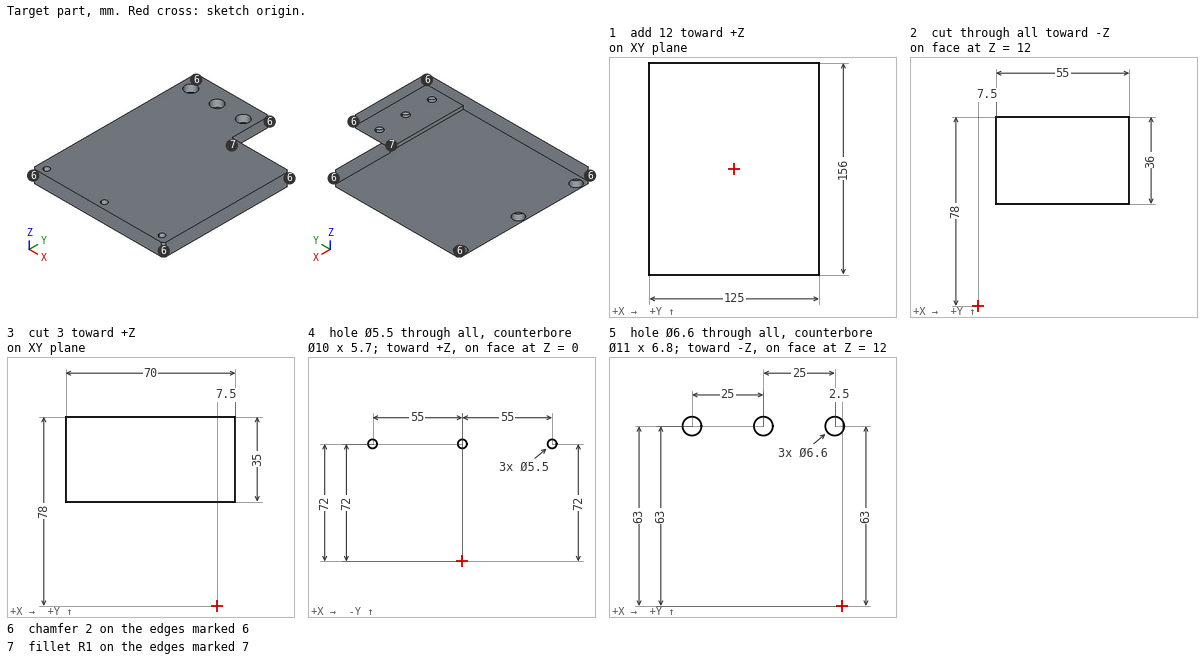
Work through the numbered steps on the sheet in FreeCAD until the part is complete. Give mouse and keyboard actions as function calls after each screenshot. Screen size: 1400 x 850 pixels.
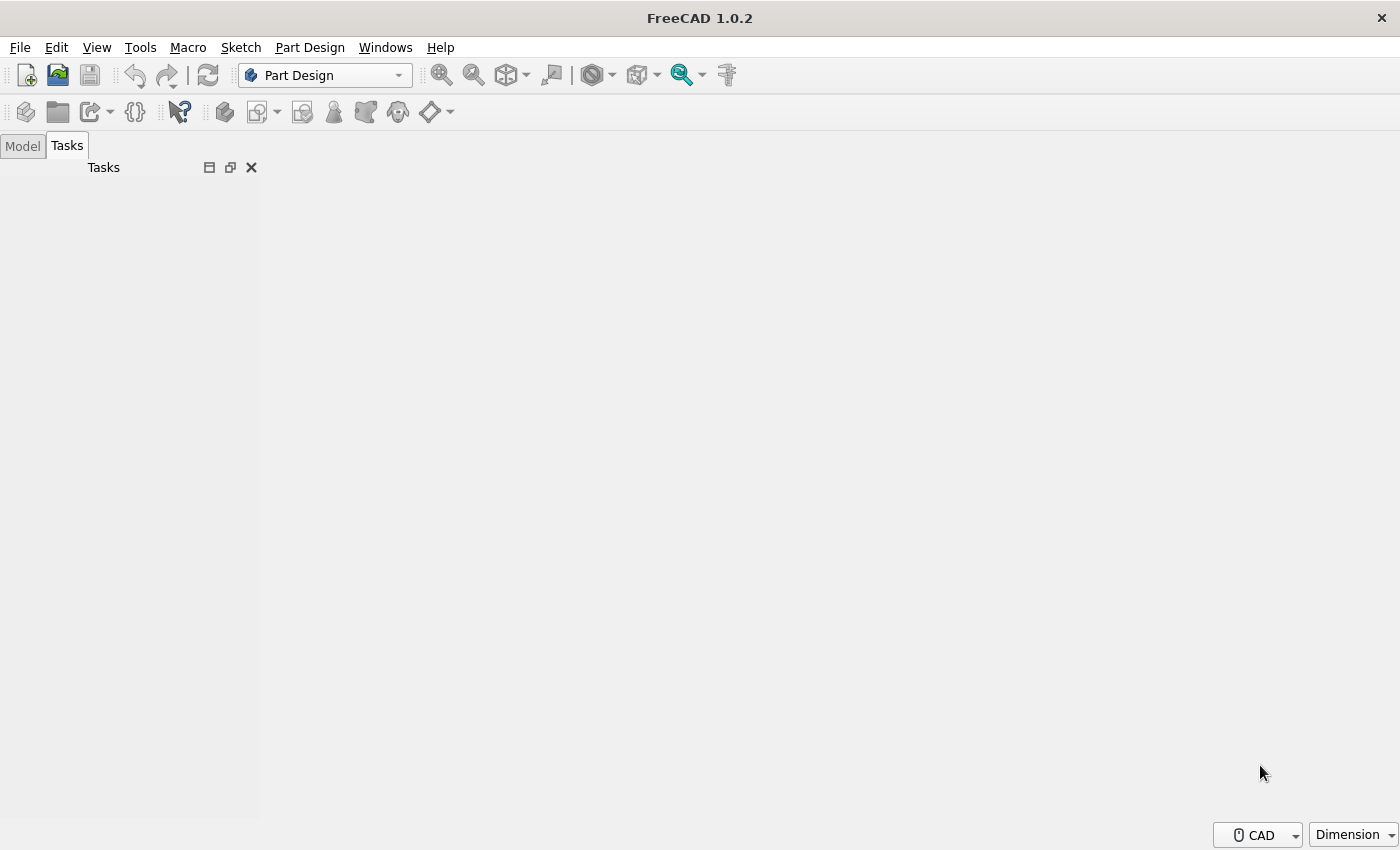
click(26, 76)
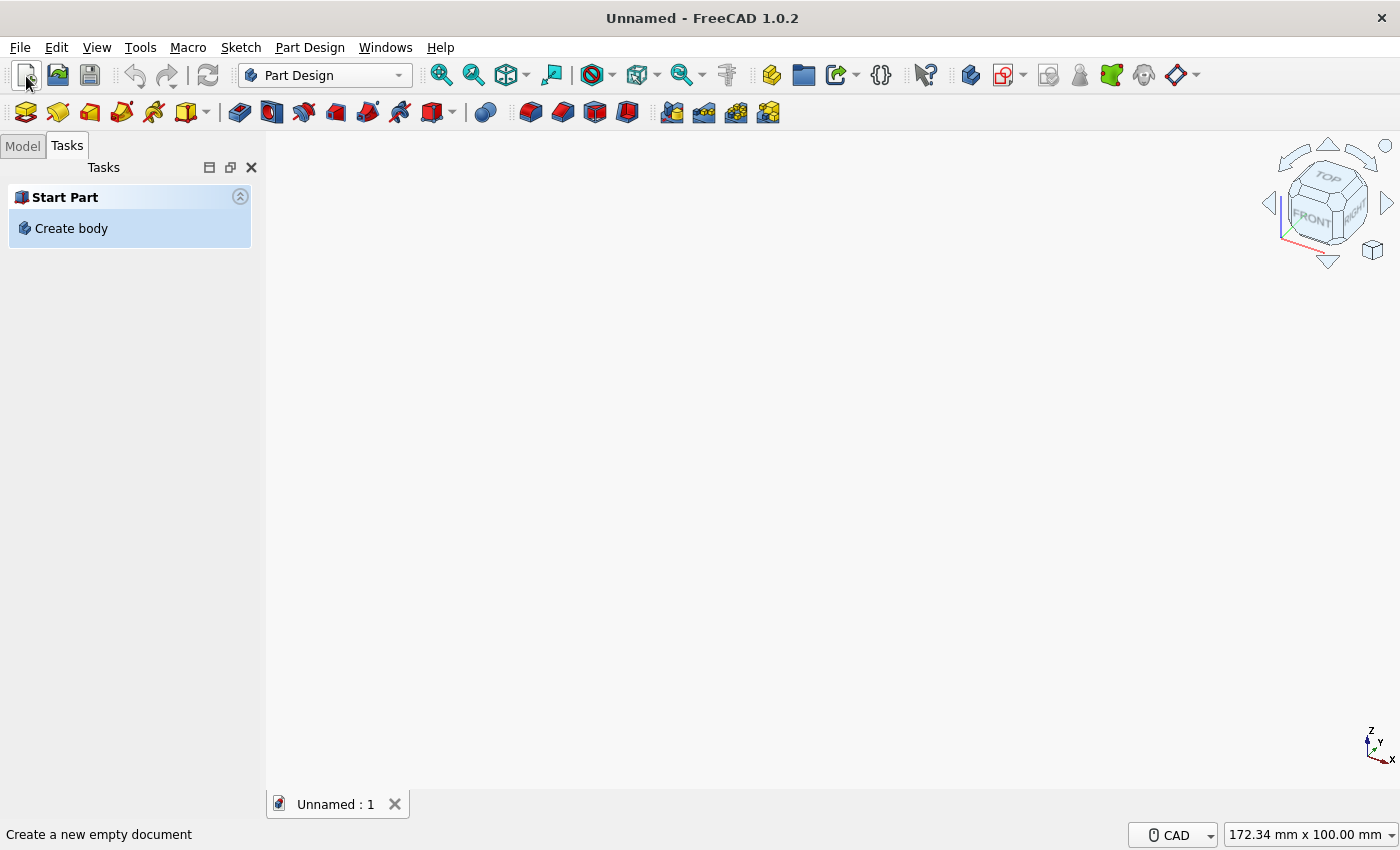
click(1004, 76)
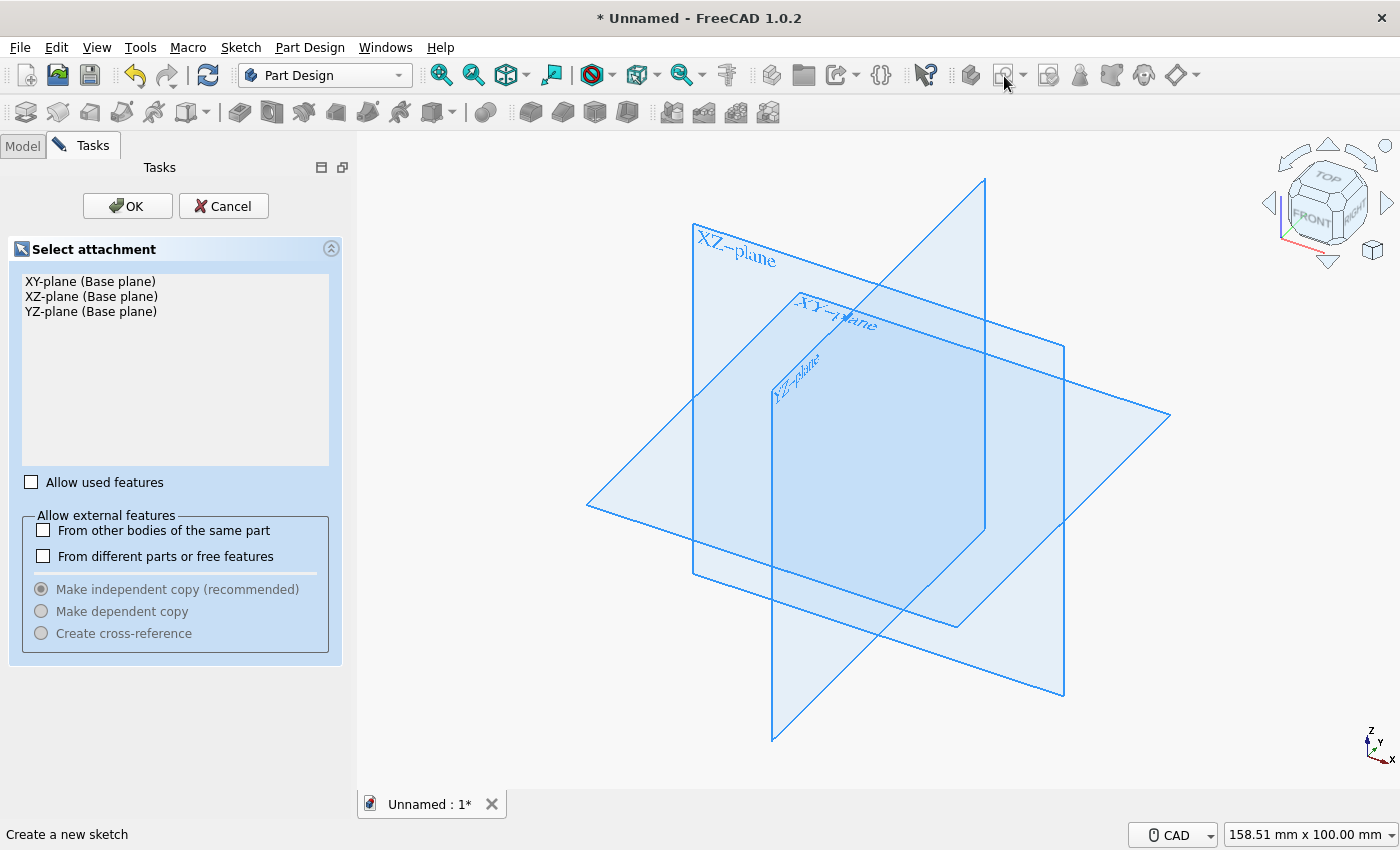
click(82, 282)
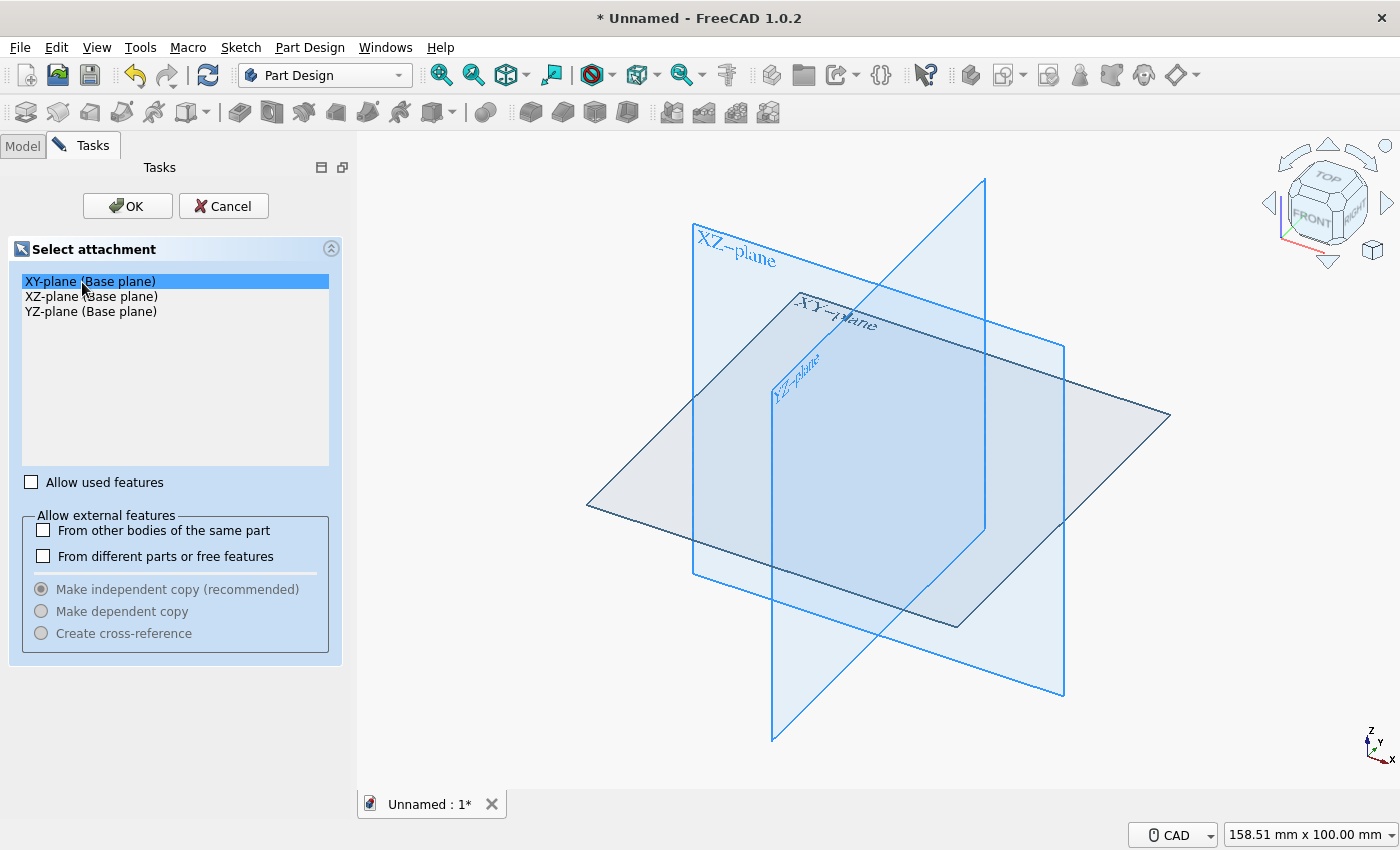
click(128, 206)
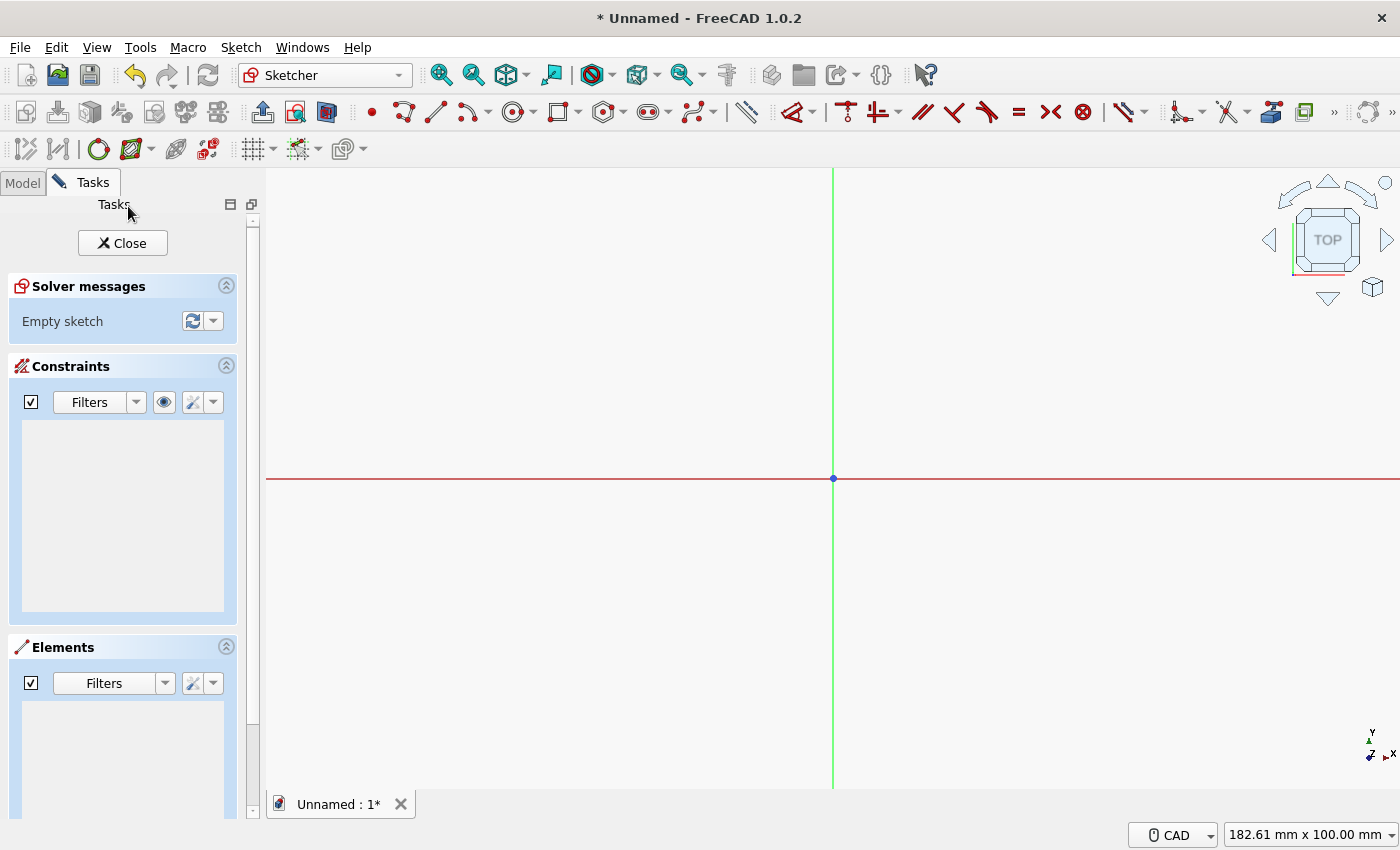
scroll(709, 478, down, 4)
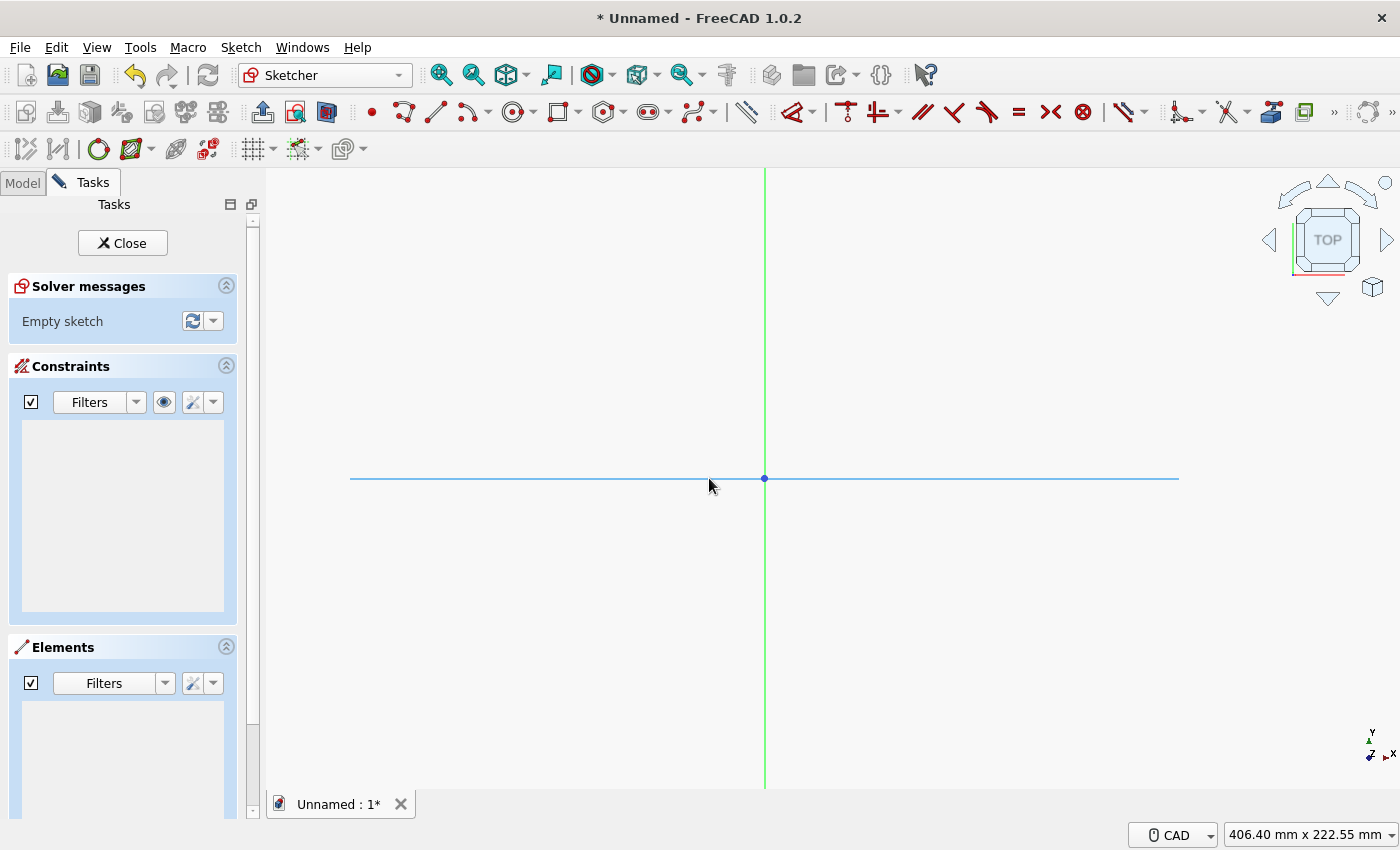
click(580, 112)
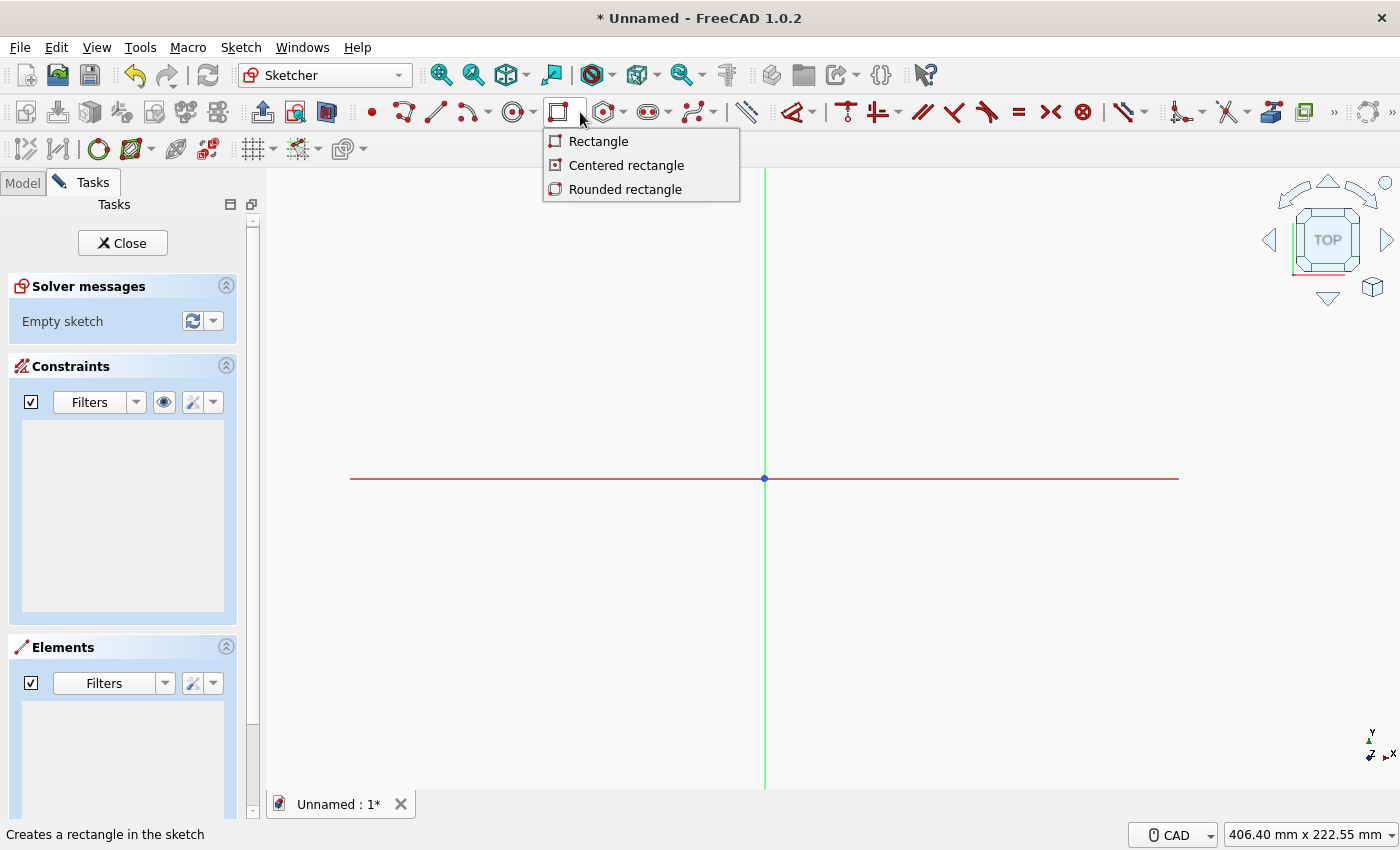
click(642, 165)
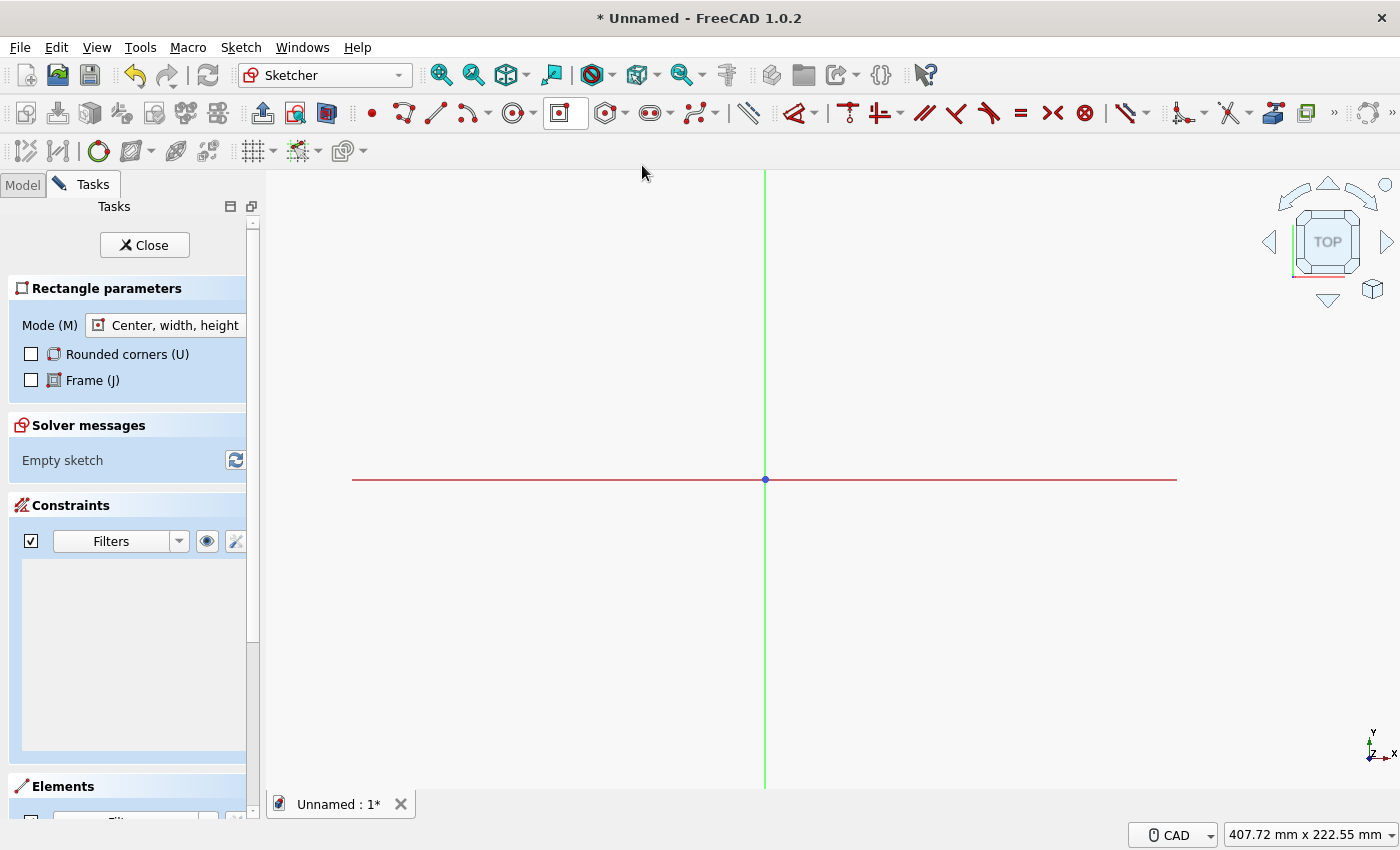
click(765, 480)
move(939, 263)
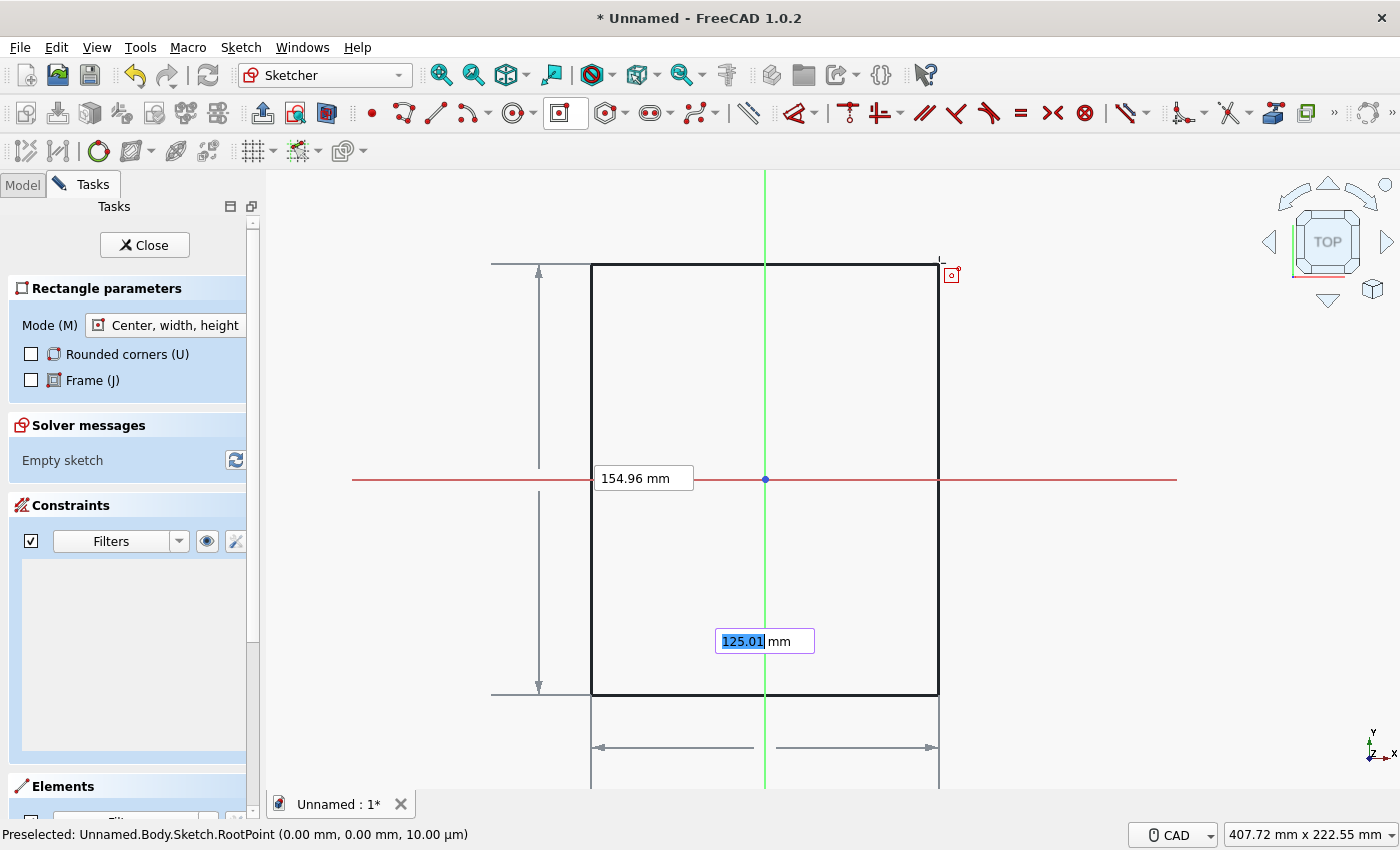
text(125)
key(Tab)
text(156)
key(Return)
key(Escape)